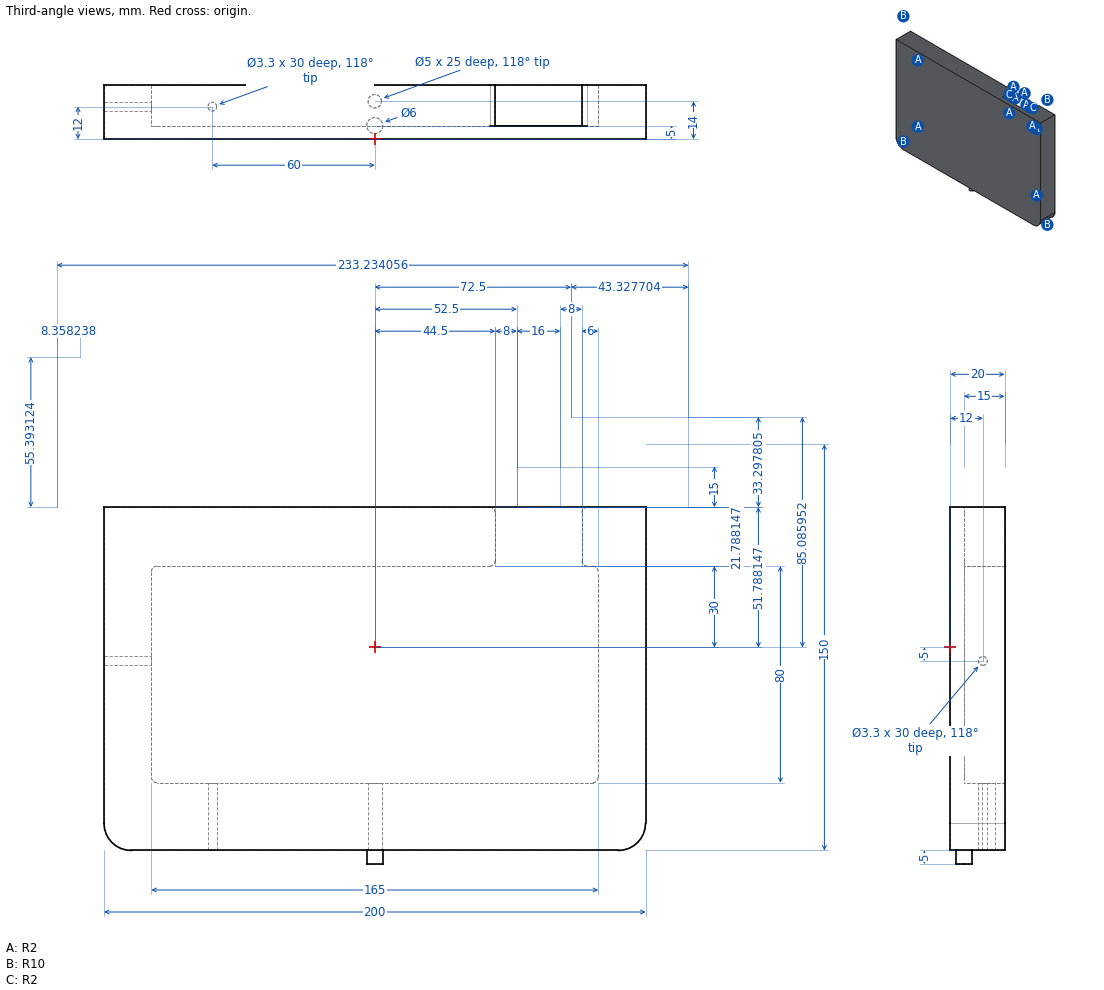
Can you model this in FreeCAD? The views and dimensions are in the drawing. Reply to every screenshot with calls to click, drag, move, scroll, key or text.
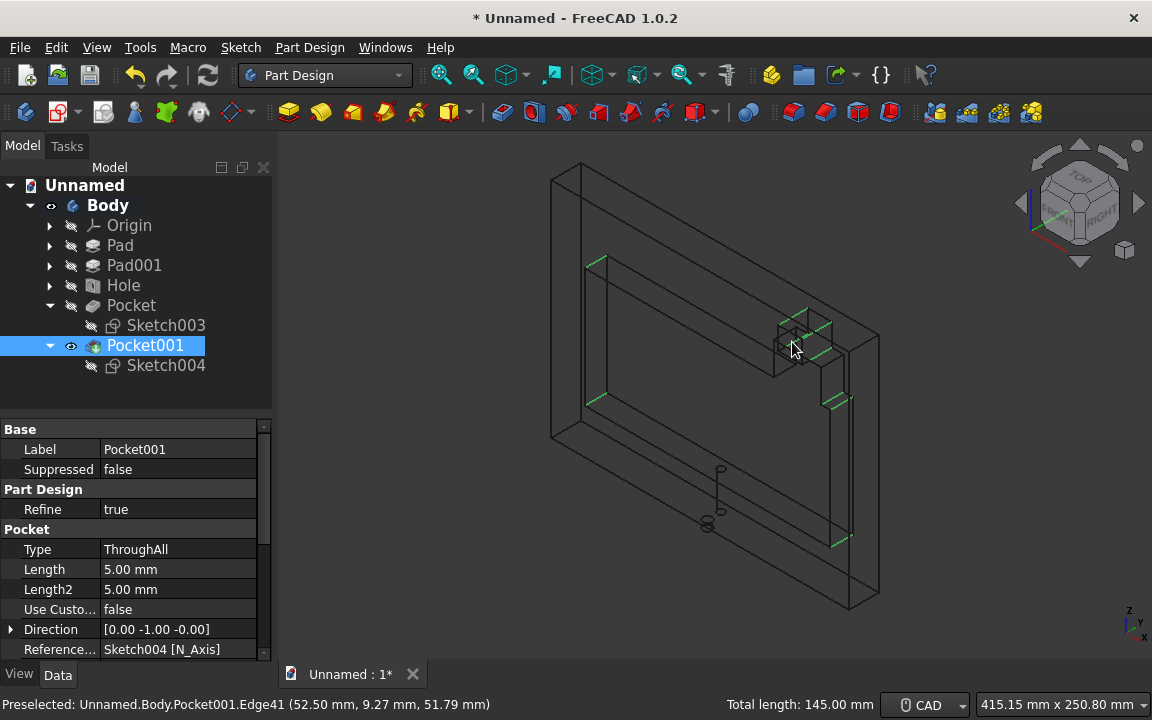
click(785, 370, ctrl)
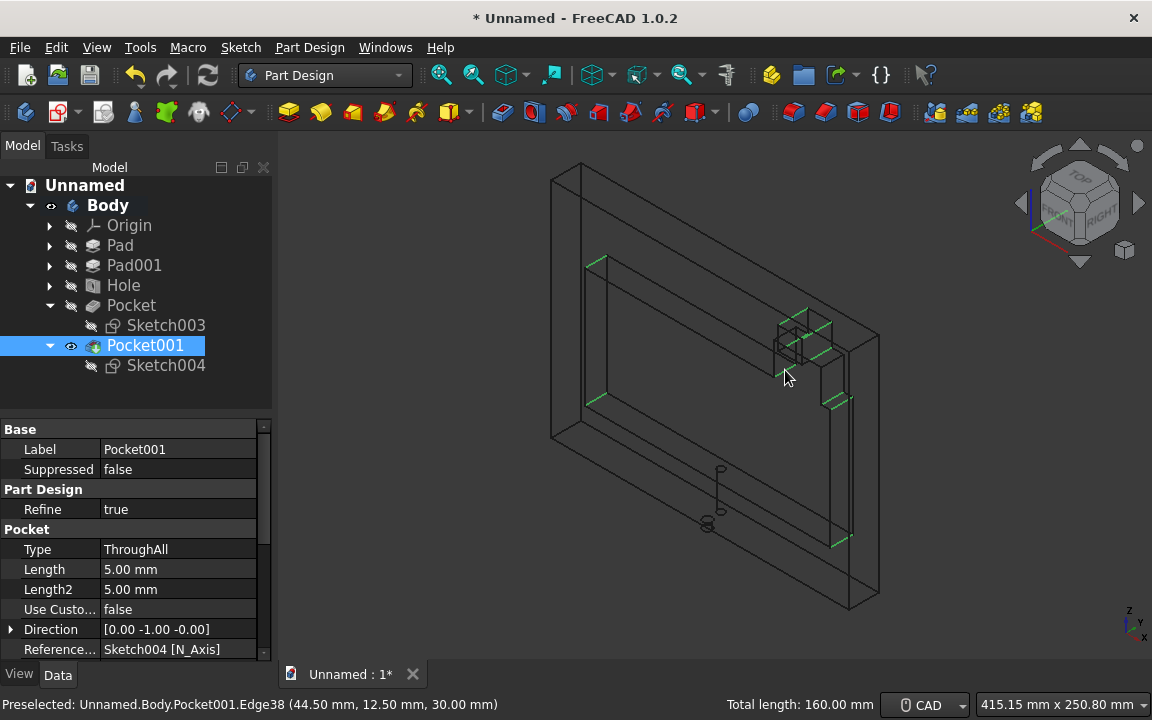
key(v)
key(1)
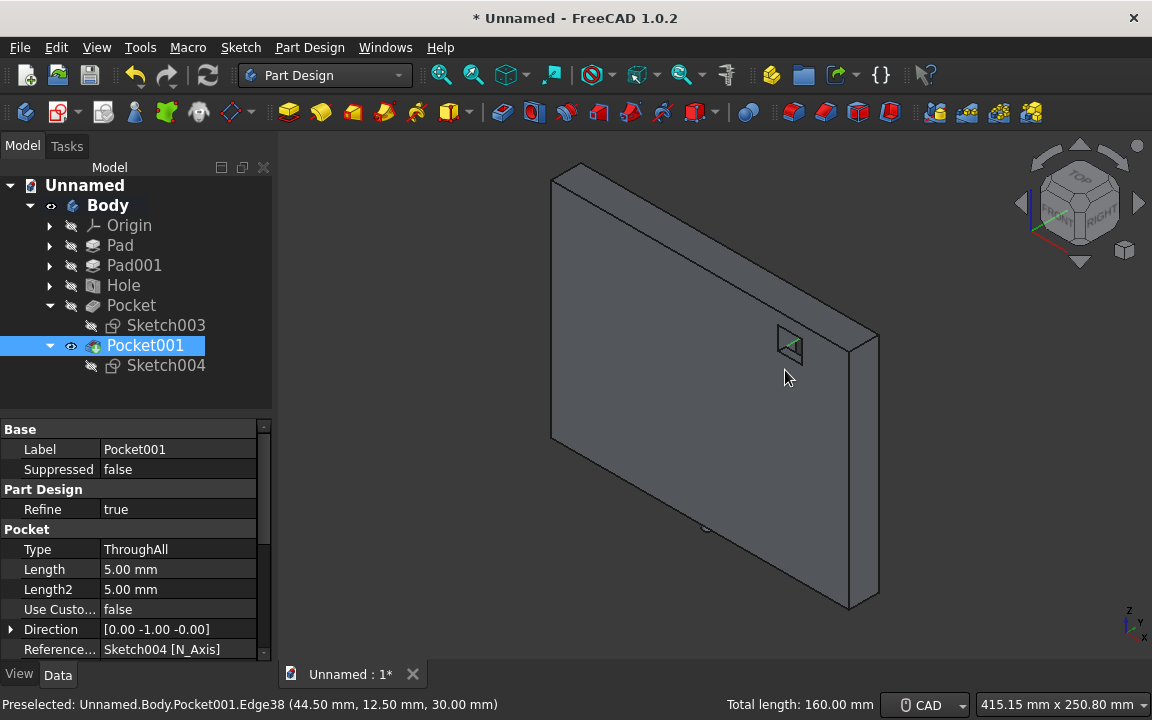
click(794, 112)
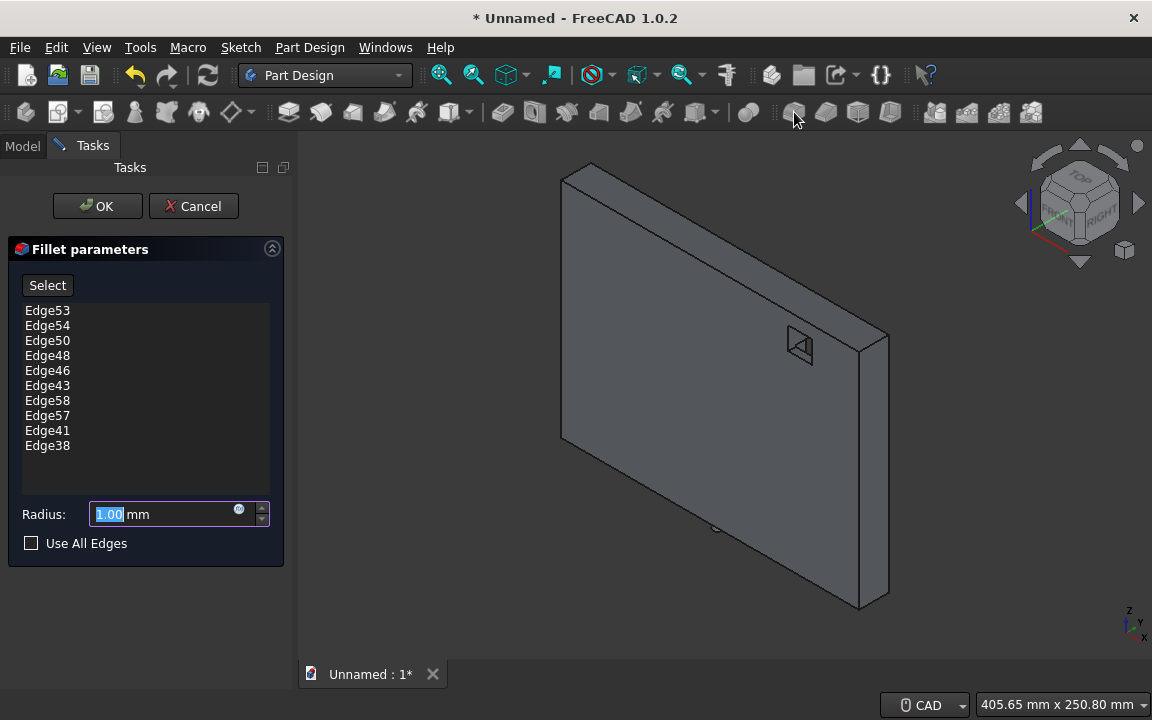
text(2)
key(Tab)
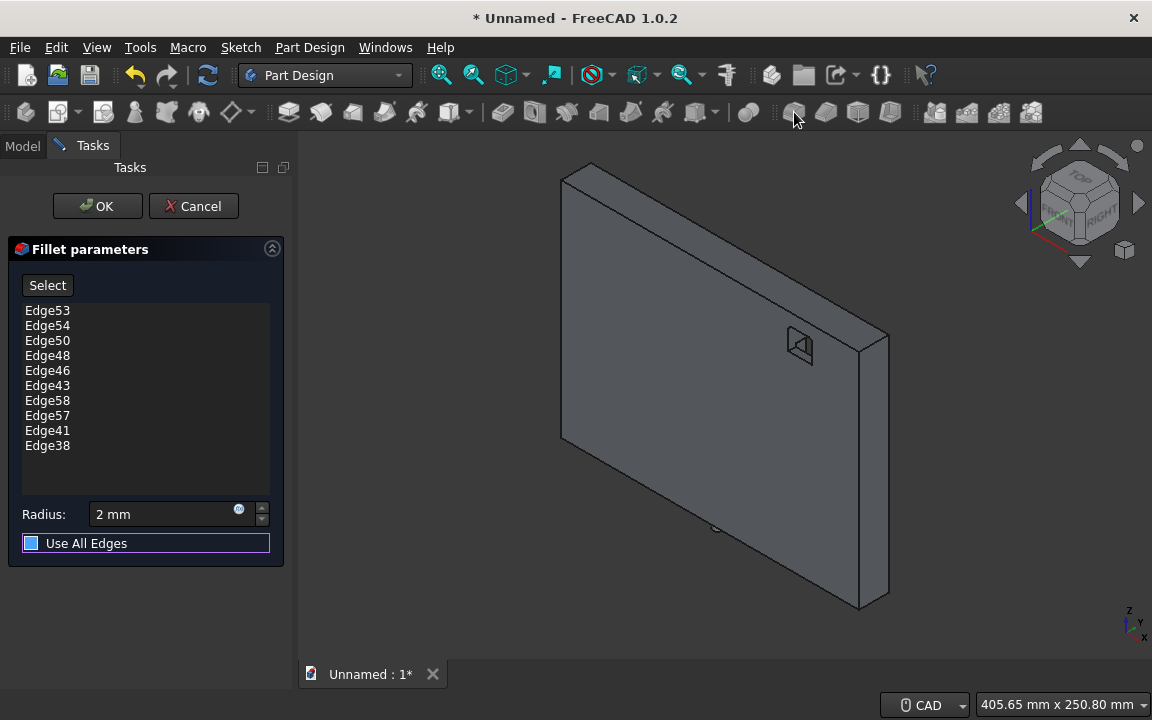
click(98, 206)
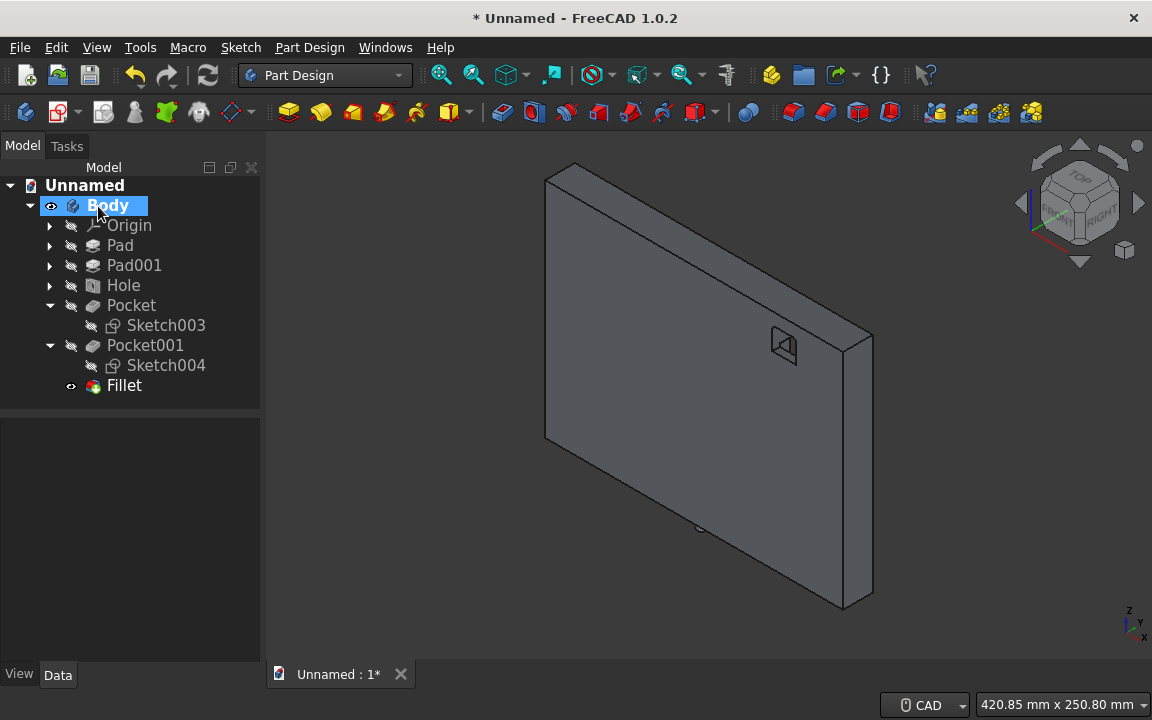
key(6)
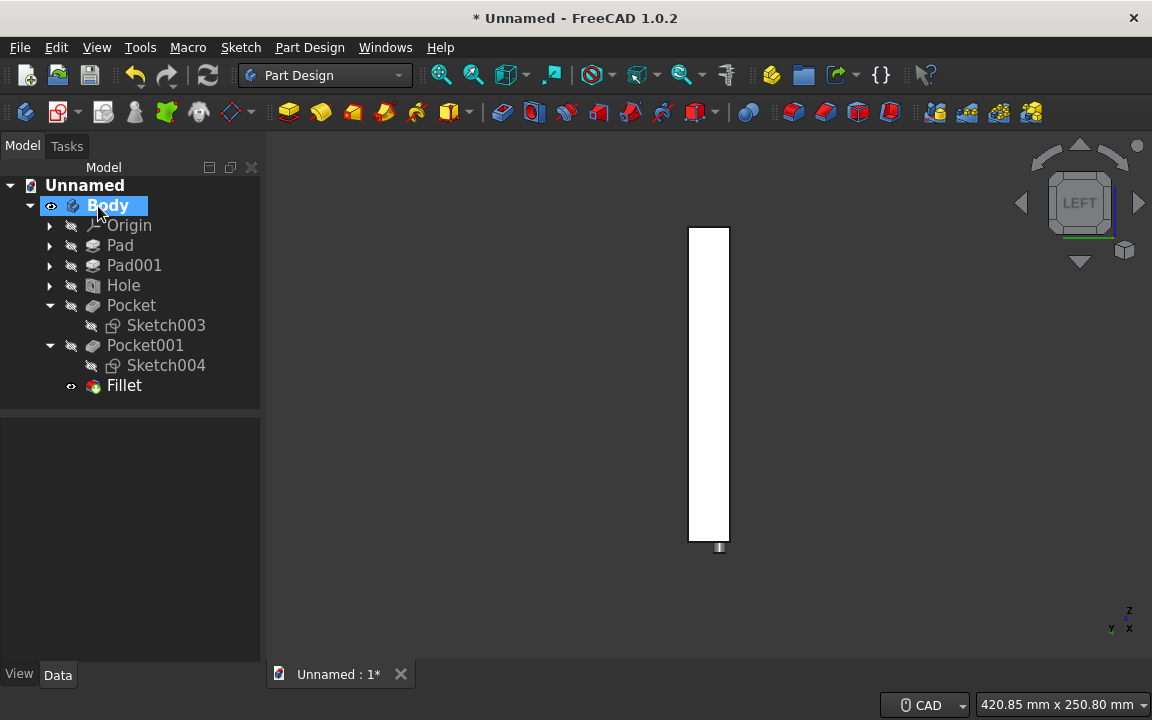
click(709, 248)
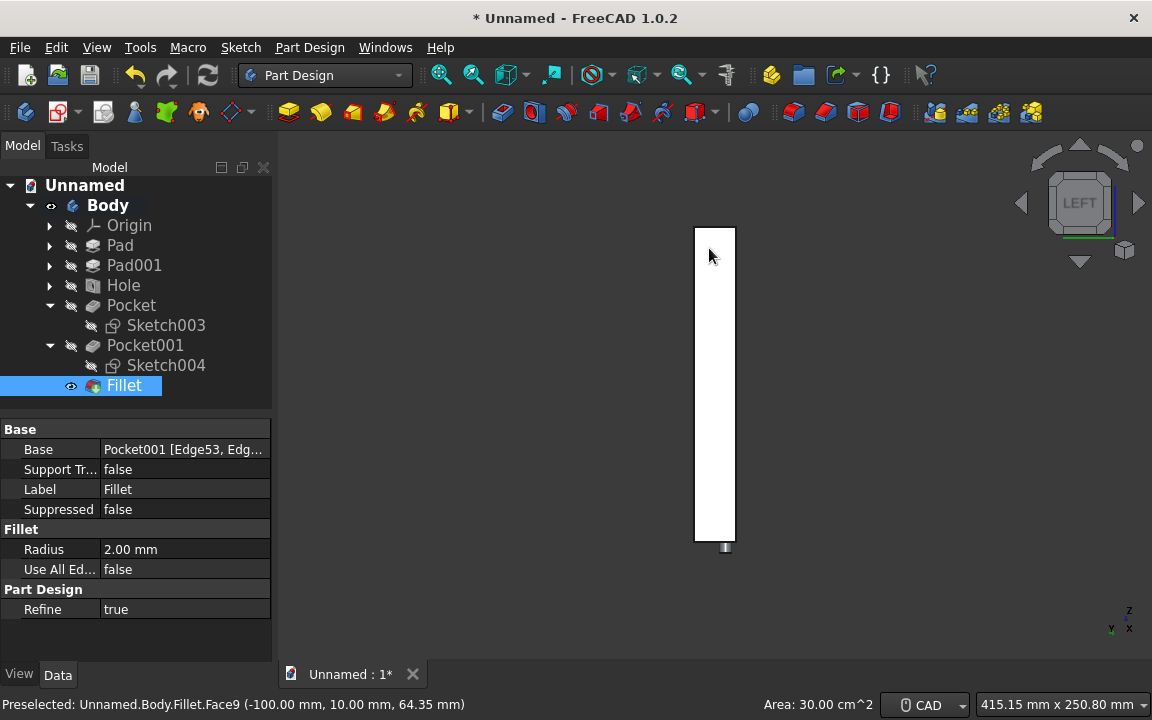
click(58, 112)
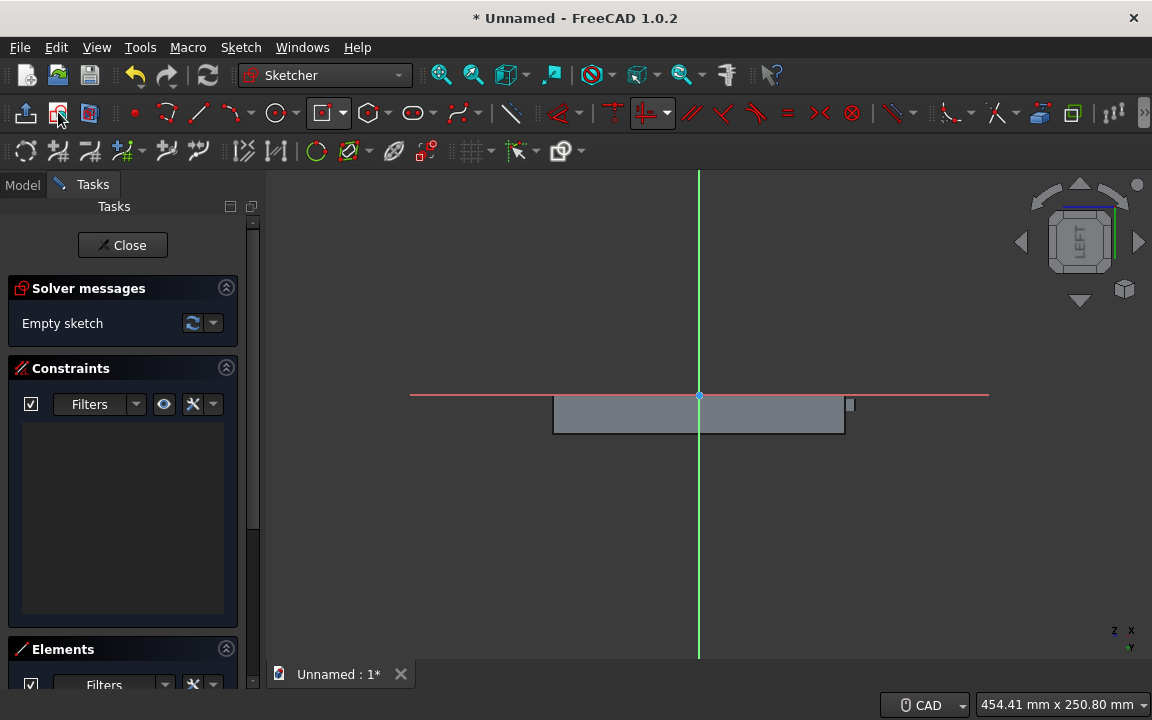
scroll(713, 419, up, 15)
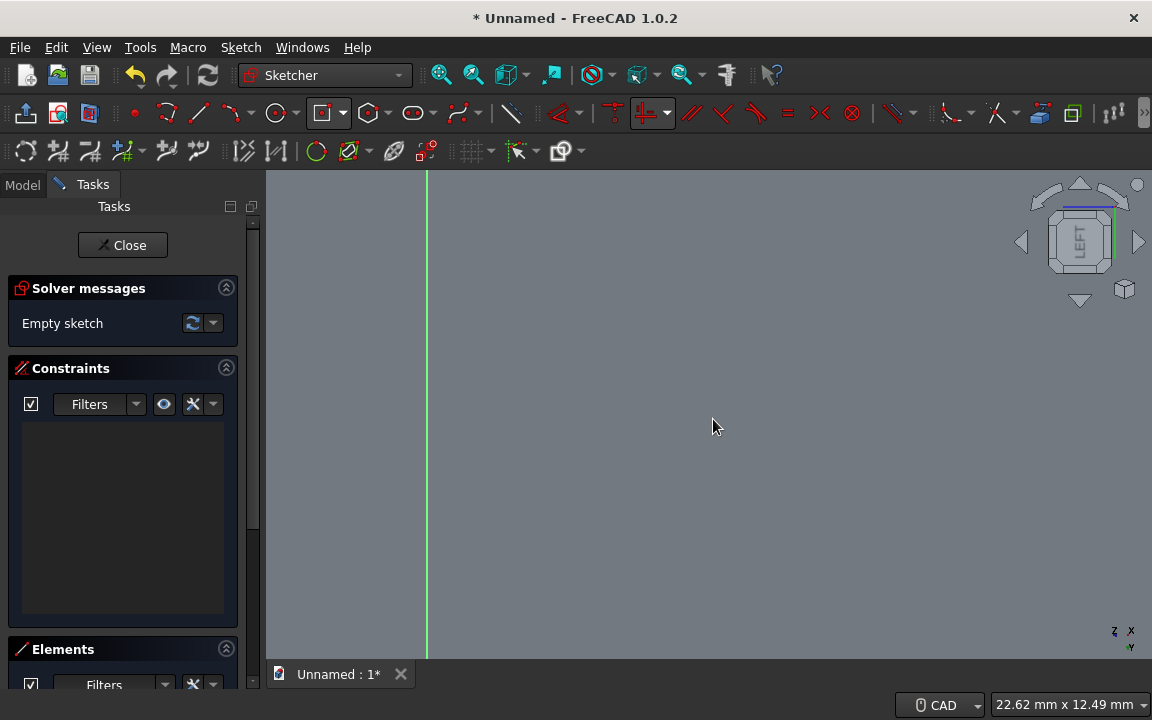
scroll(609, 383, up, 4)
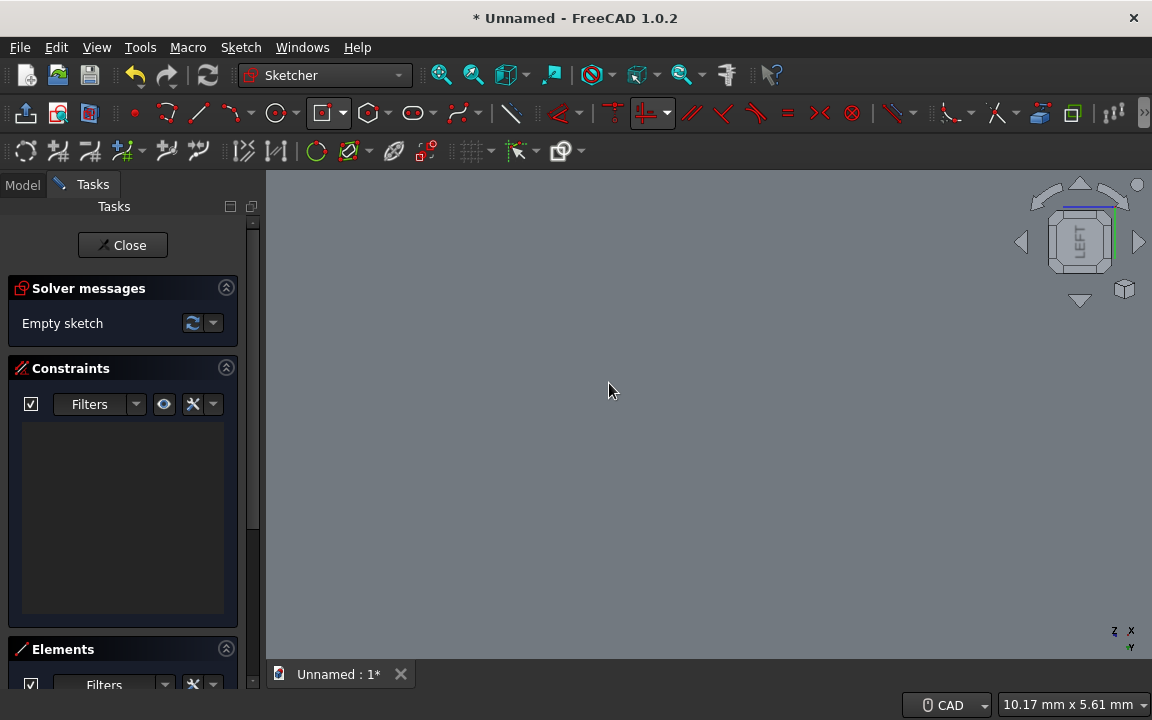
click(276, 114)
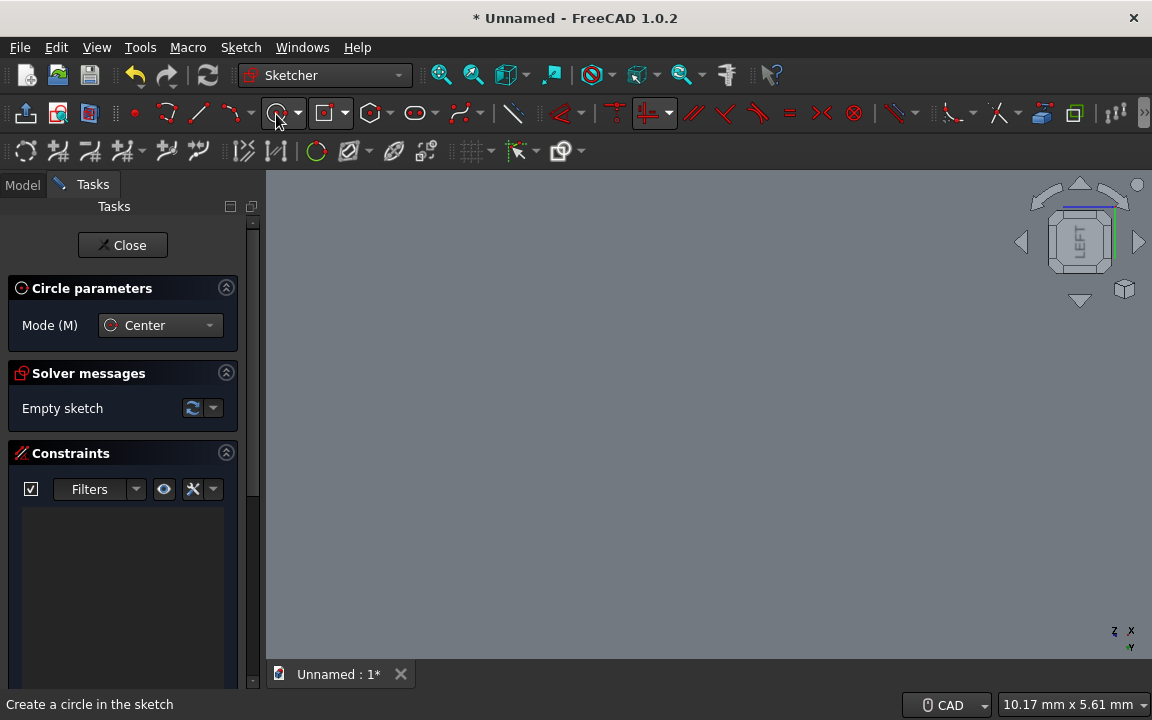
click(640, 414)
click(741, 312)
key(Escape)